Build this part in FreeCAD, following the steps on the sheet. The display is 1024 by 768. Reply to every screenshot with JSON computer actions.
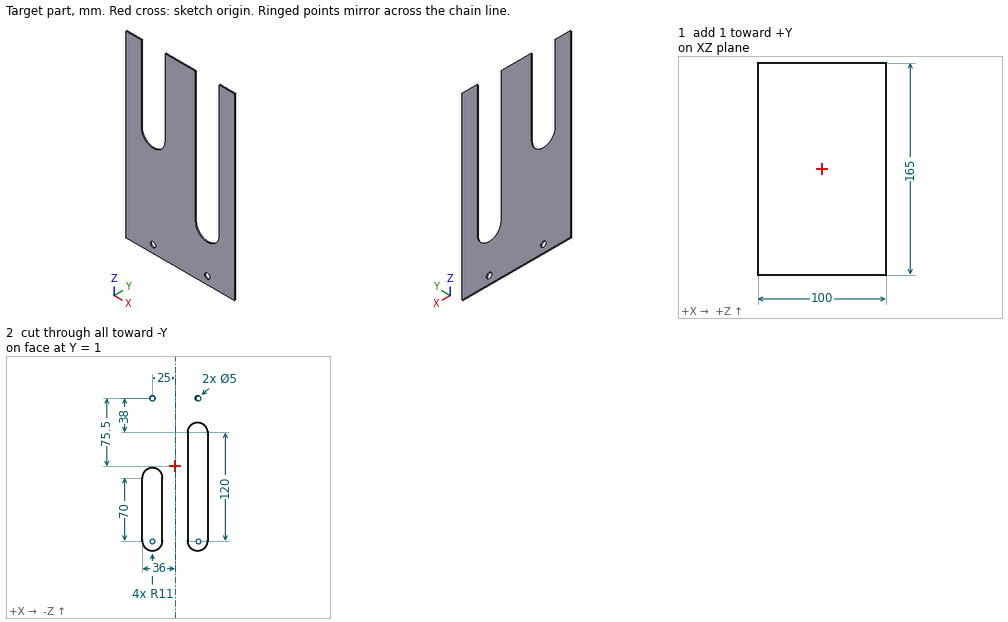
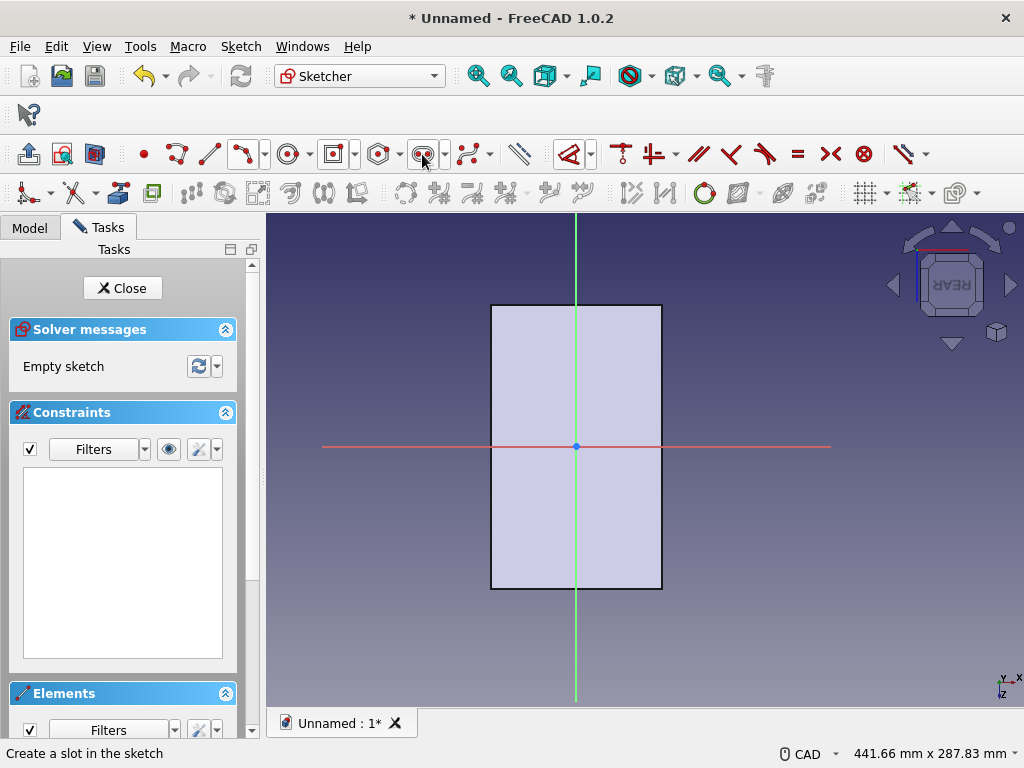
{"action": "left_click", "coordinate": [534, 589]}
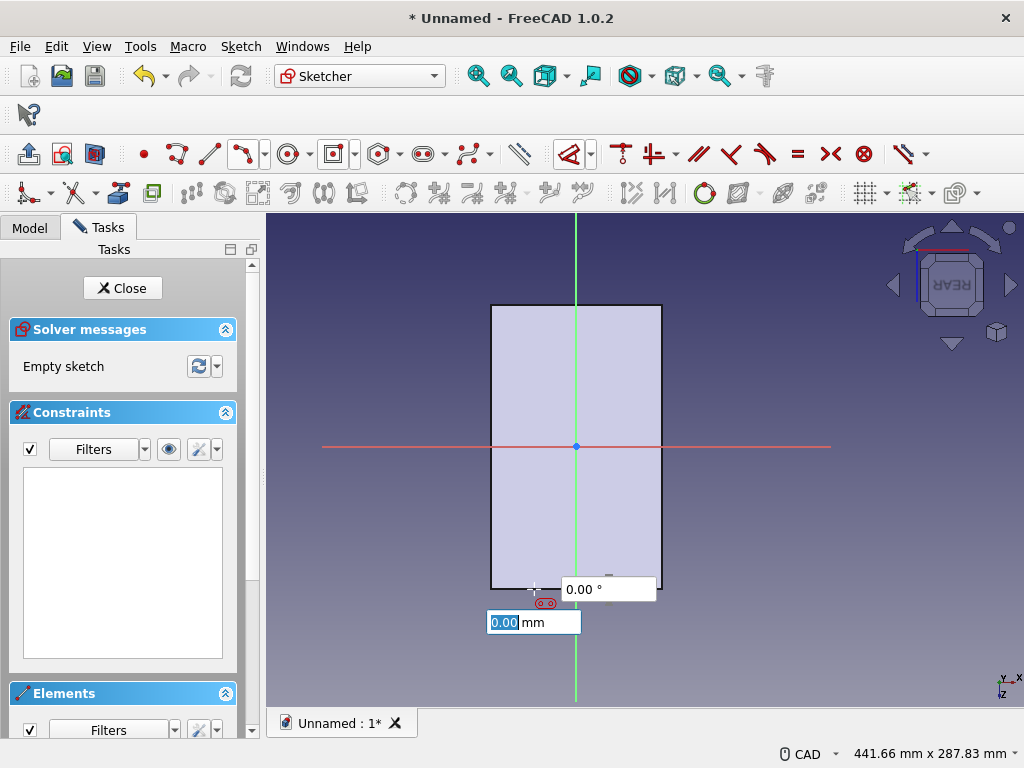
{"action": "left_click", "coordinate": [534, 468]}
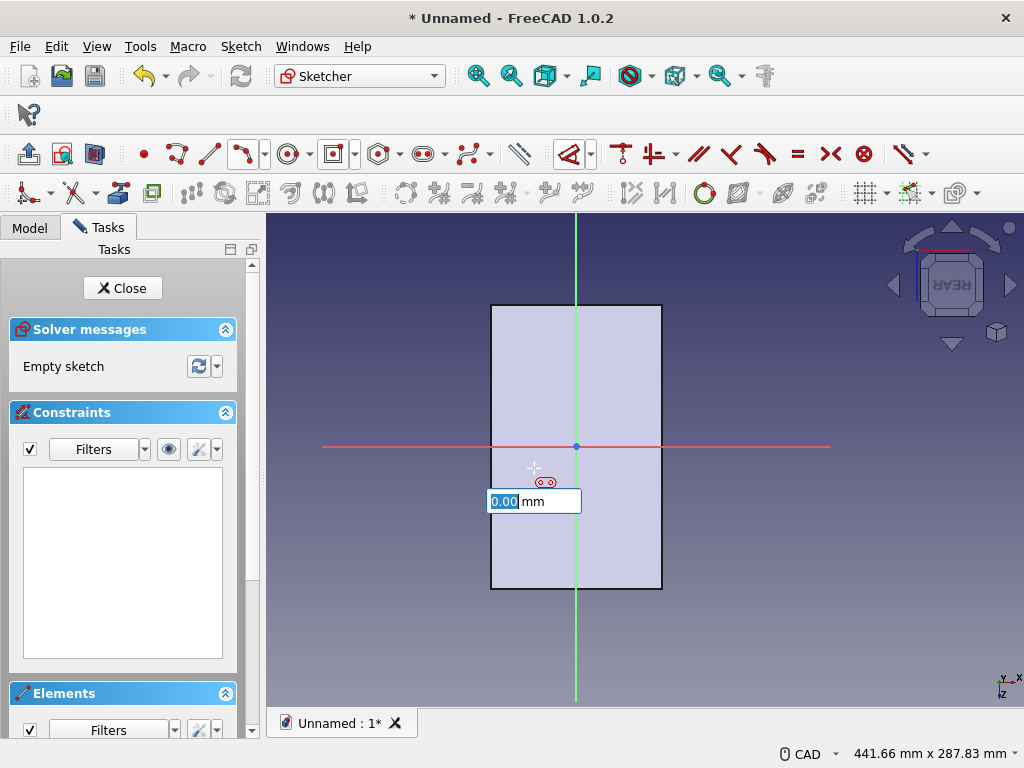
{"action": "left_click", "coordinate": [515, 528]}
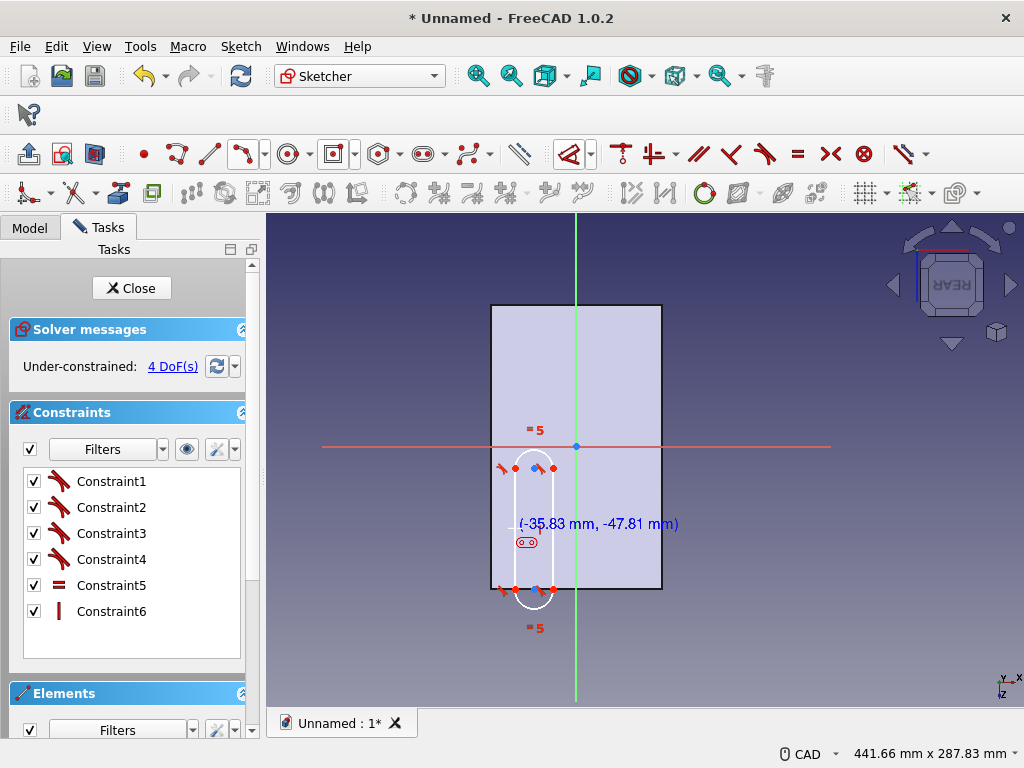
{"action": "left_click", "coordinate": [619, 589]}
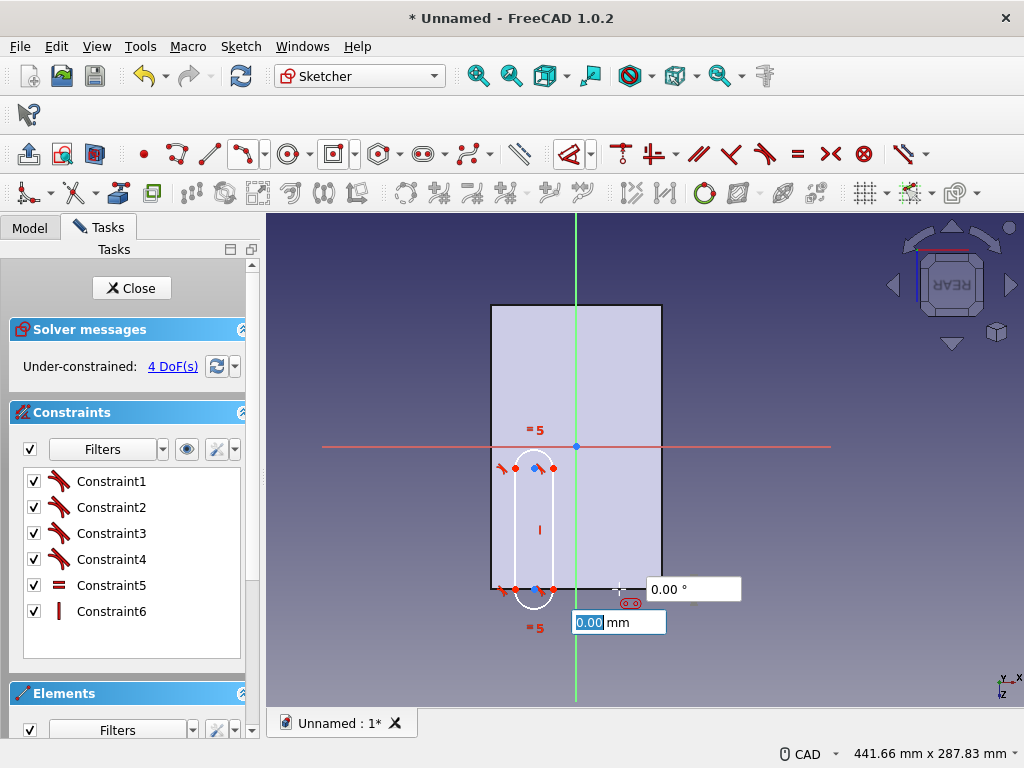
{"action": "left_click", "coordinate": [619, 383]}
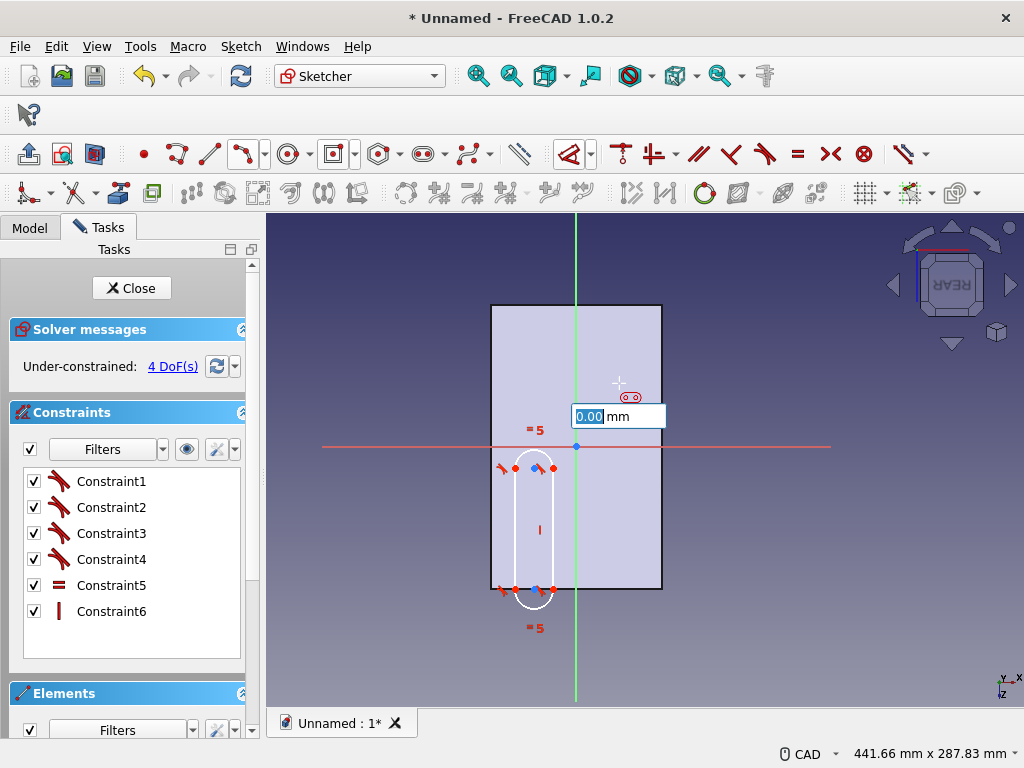
{"action": "left_click", "coordinate": [601, 486]}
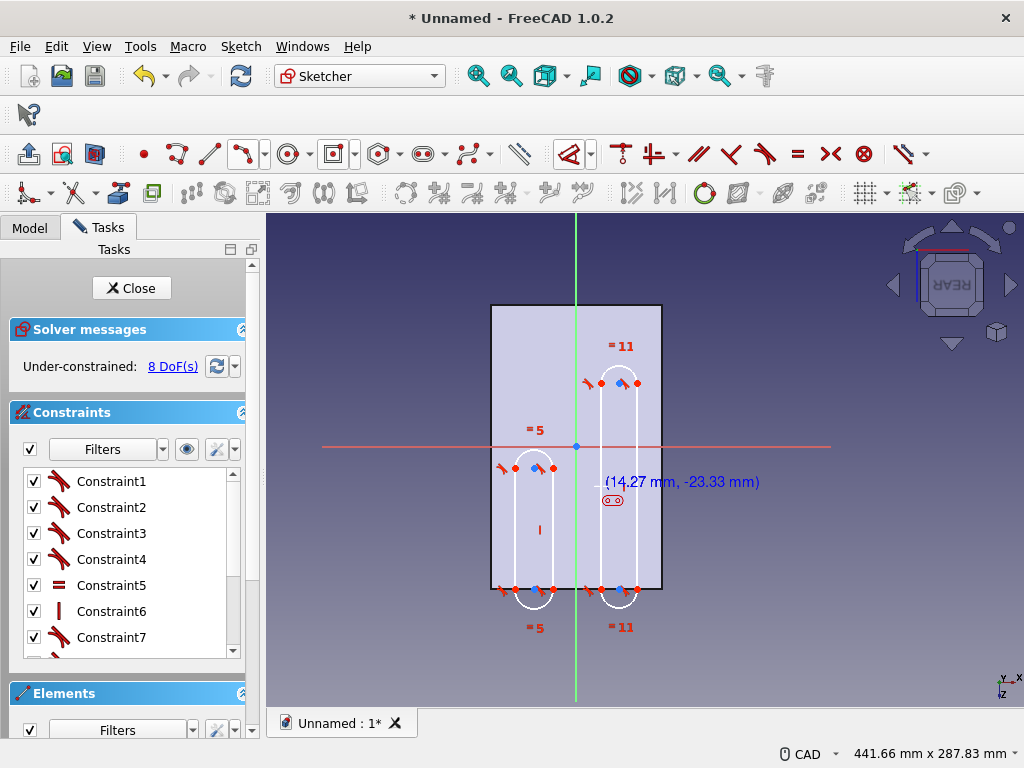
{"action": "left_click", "coordinate": [288, 154]}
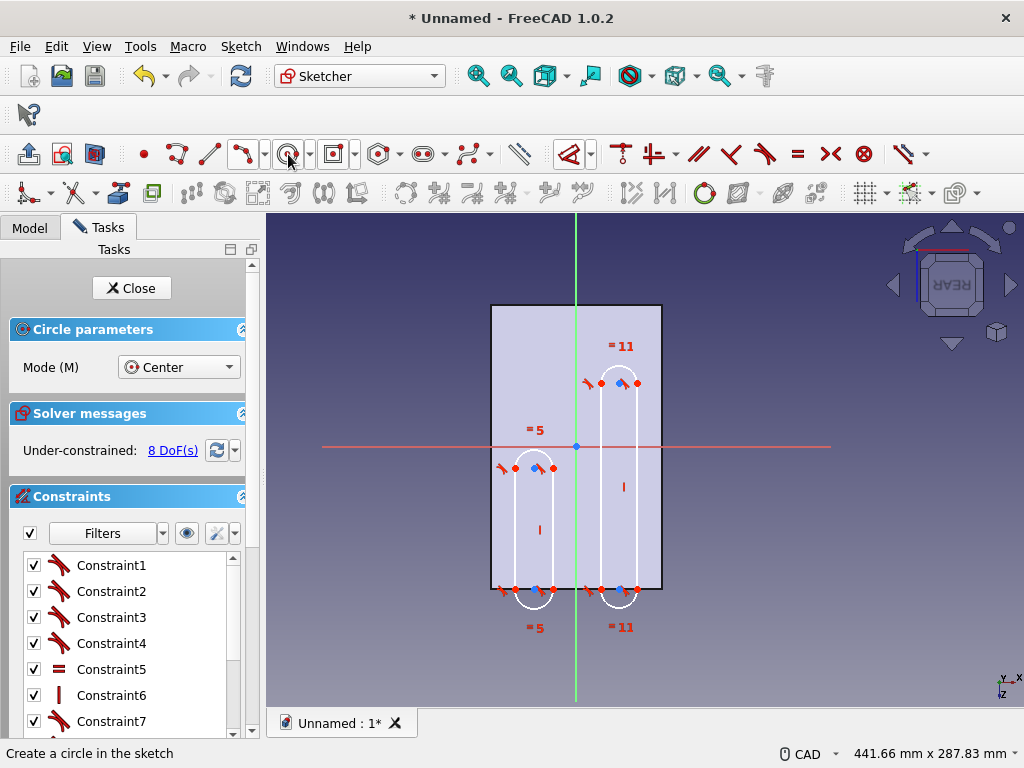
{"action": "scroll", "coordinate": [534, 317], "scroll_direction": "up", "scroll_amount": 9}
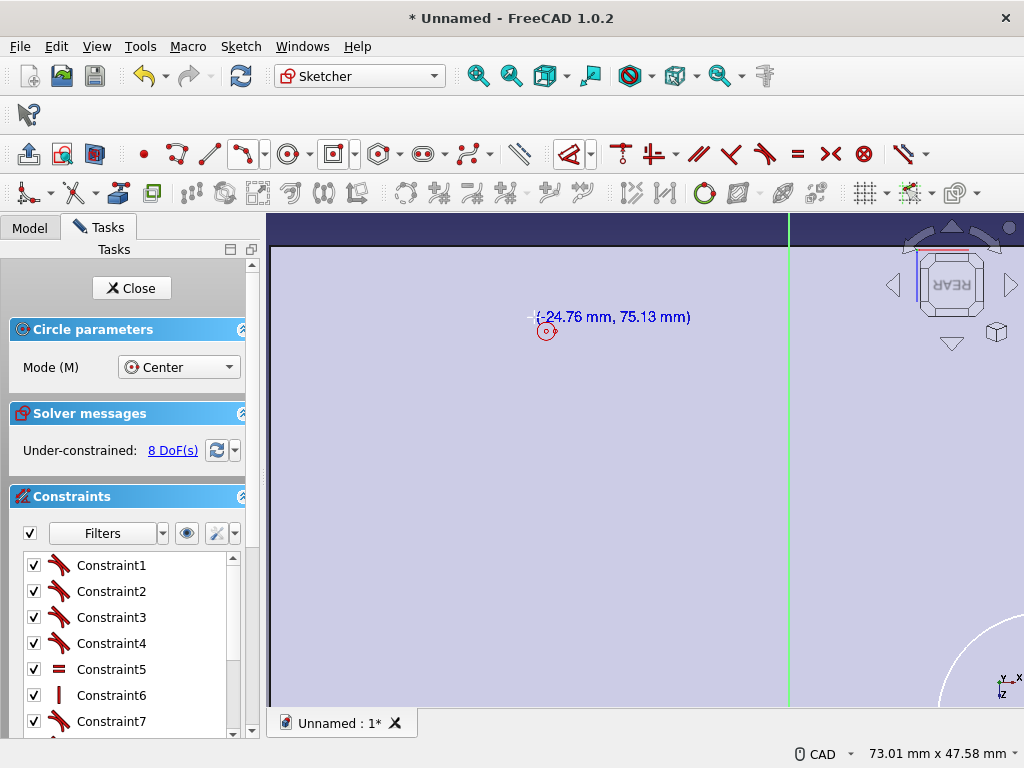
{"action": "scroll", "coordinate": [534, 317], "scroll_direction": "down", "scroll_amount": 9}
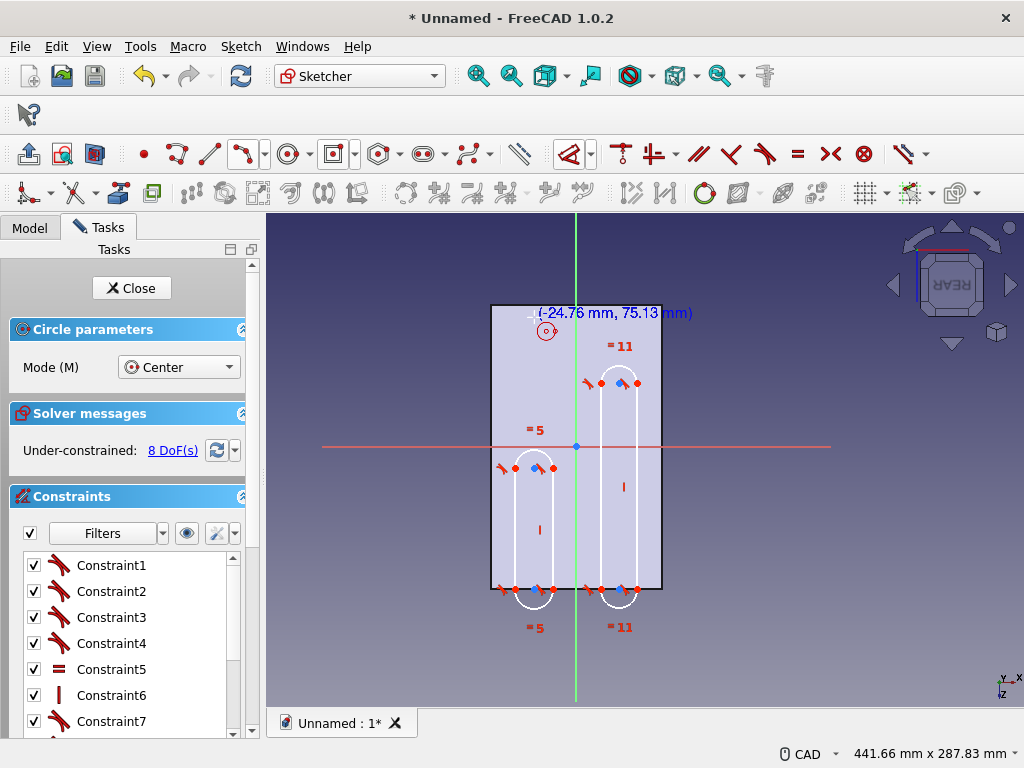
{"action": "left_click", "coordinate": [534, 317]}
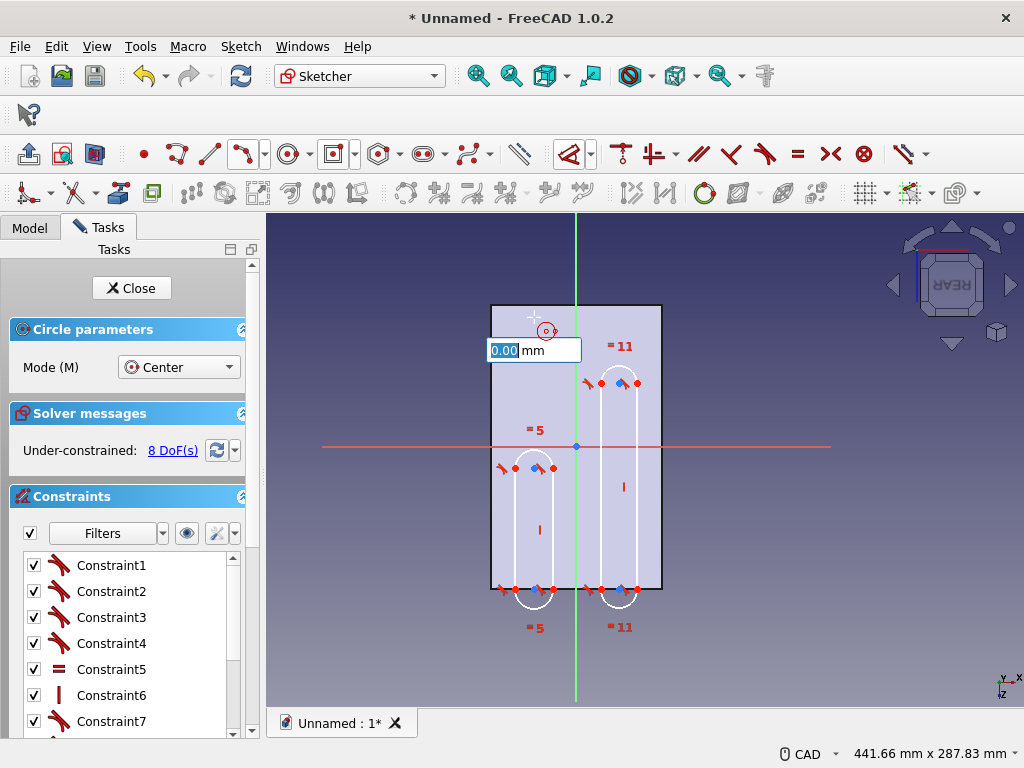
{"action": "scroll", "coordinate": [537, 314], "scroll_direction": "up", "scroll_amount": 7}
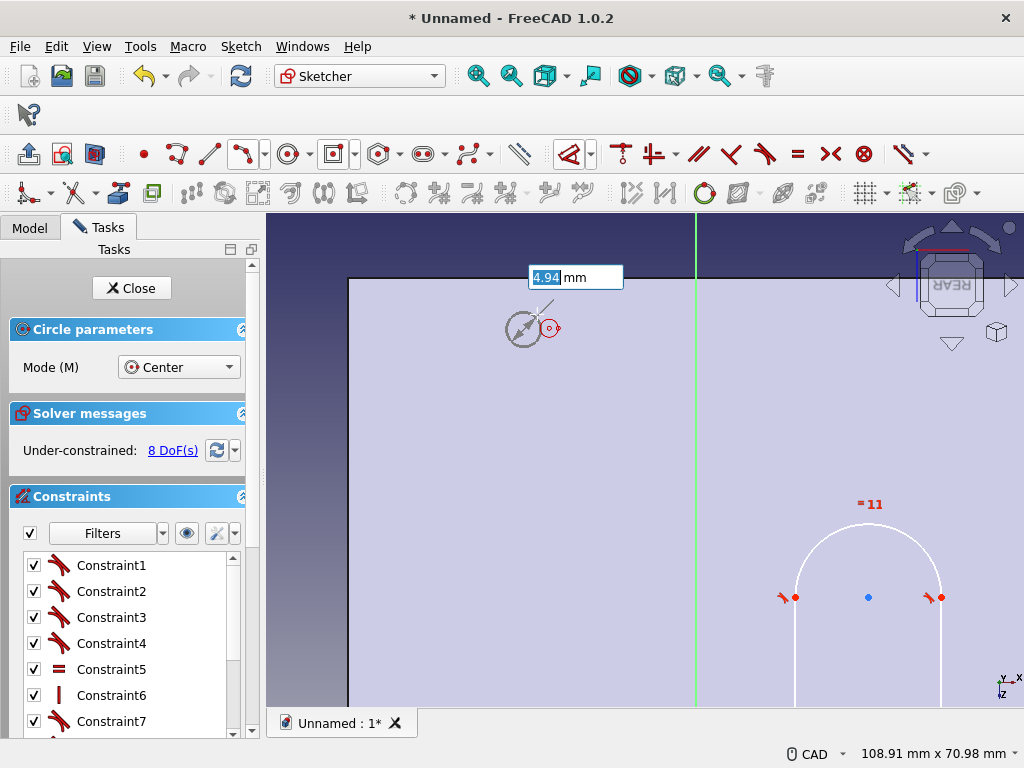
{"action": "left_click", "coordinate": [534, 315]}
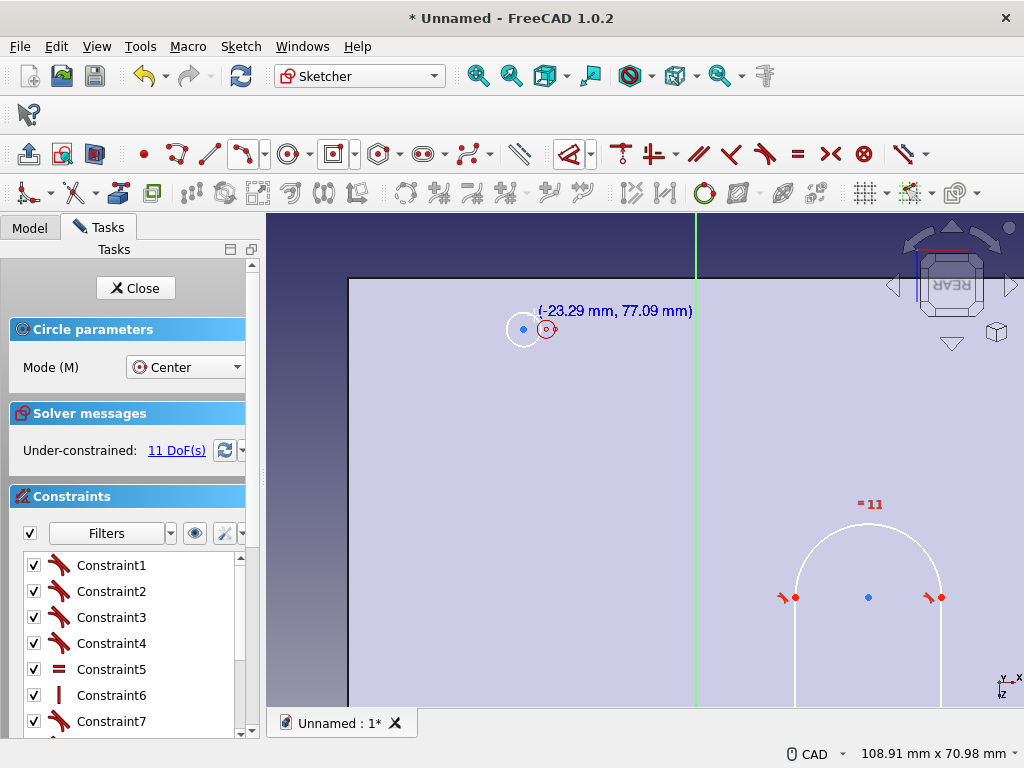
{"action": "scroll", "coordinate": [537, 314], "scroll_direction": "down", "scroll_amount": 7}